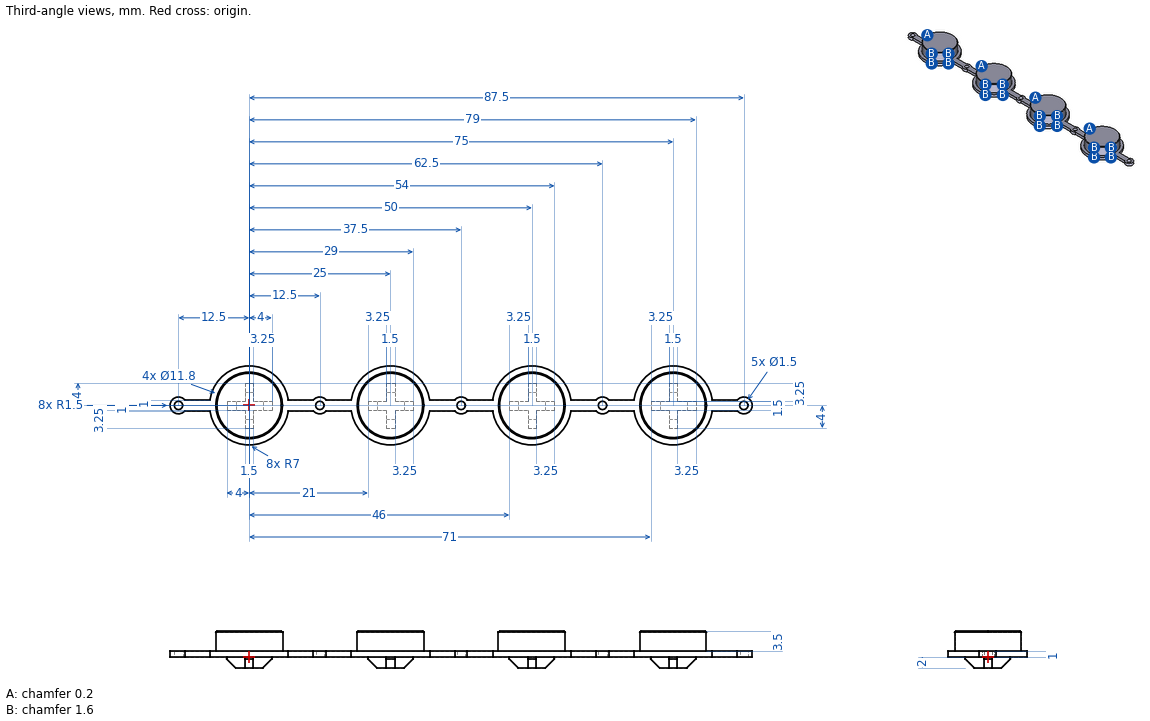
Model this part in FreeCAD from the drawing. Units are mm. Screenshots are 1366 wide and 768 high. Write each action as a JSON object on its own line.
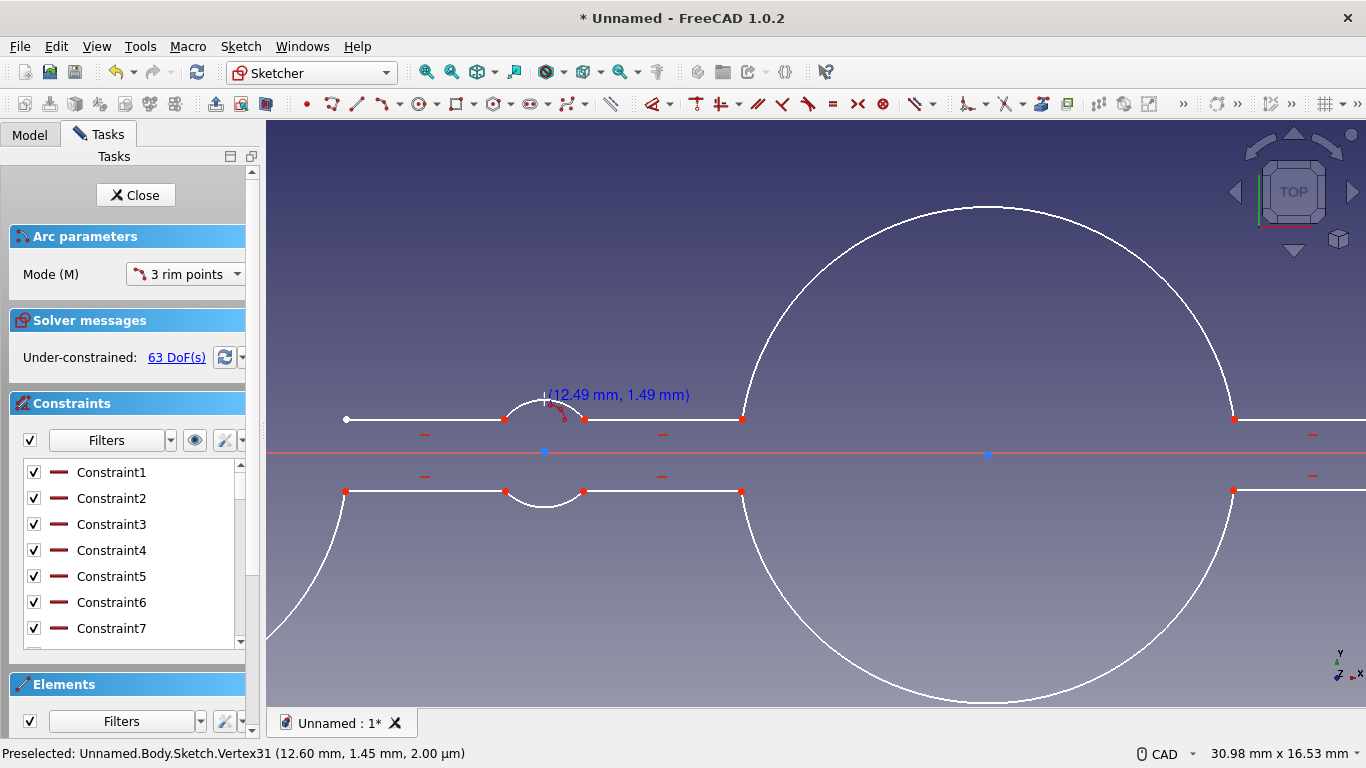
{"action": "left_click", "coordinate": [346, 420]}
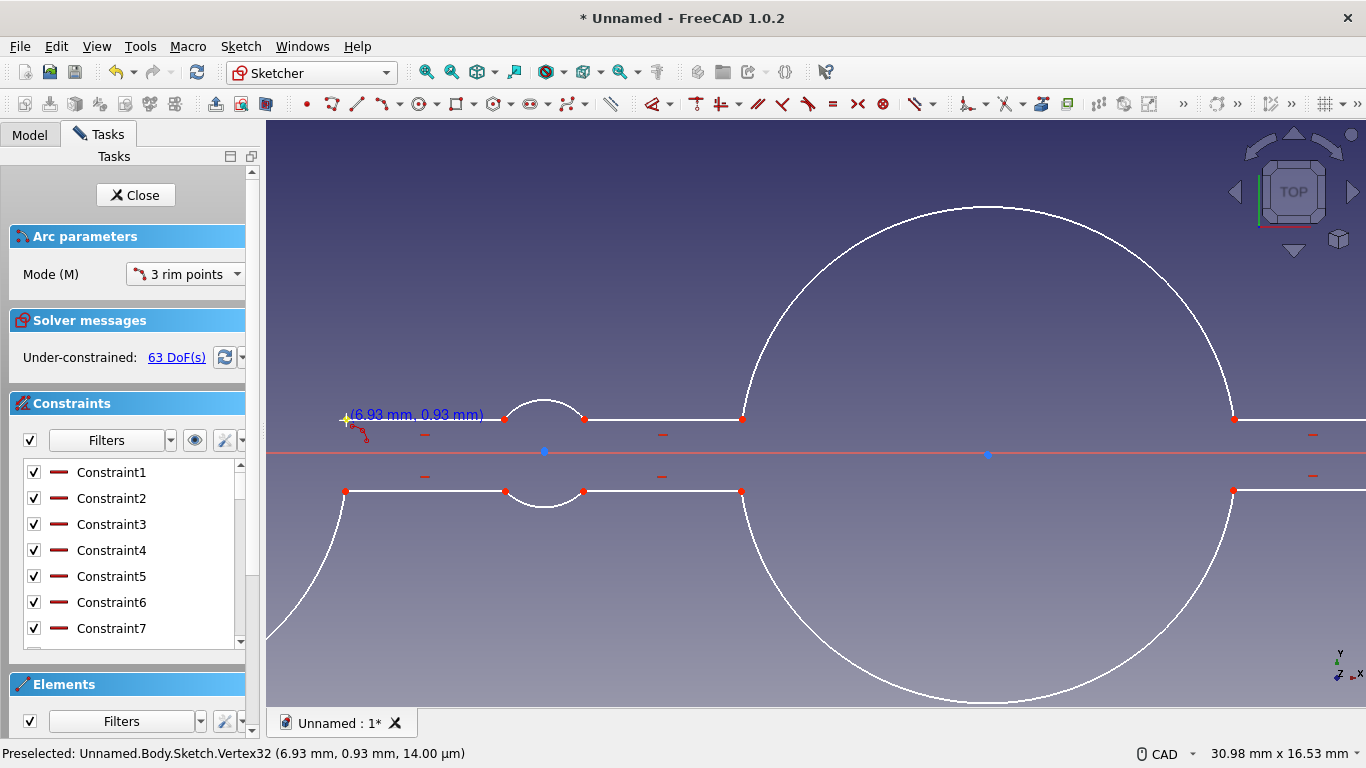
{"action": "scroll", "coordinate": [612, 406], "scroll_direction": "down", "scroll_amount": 9}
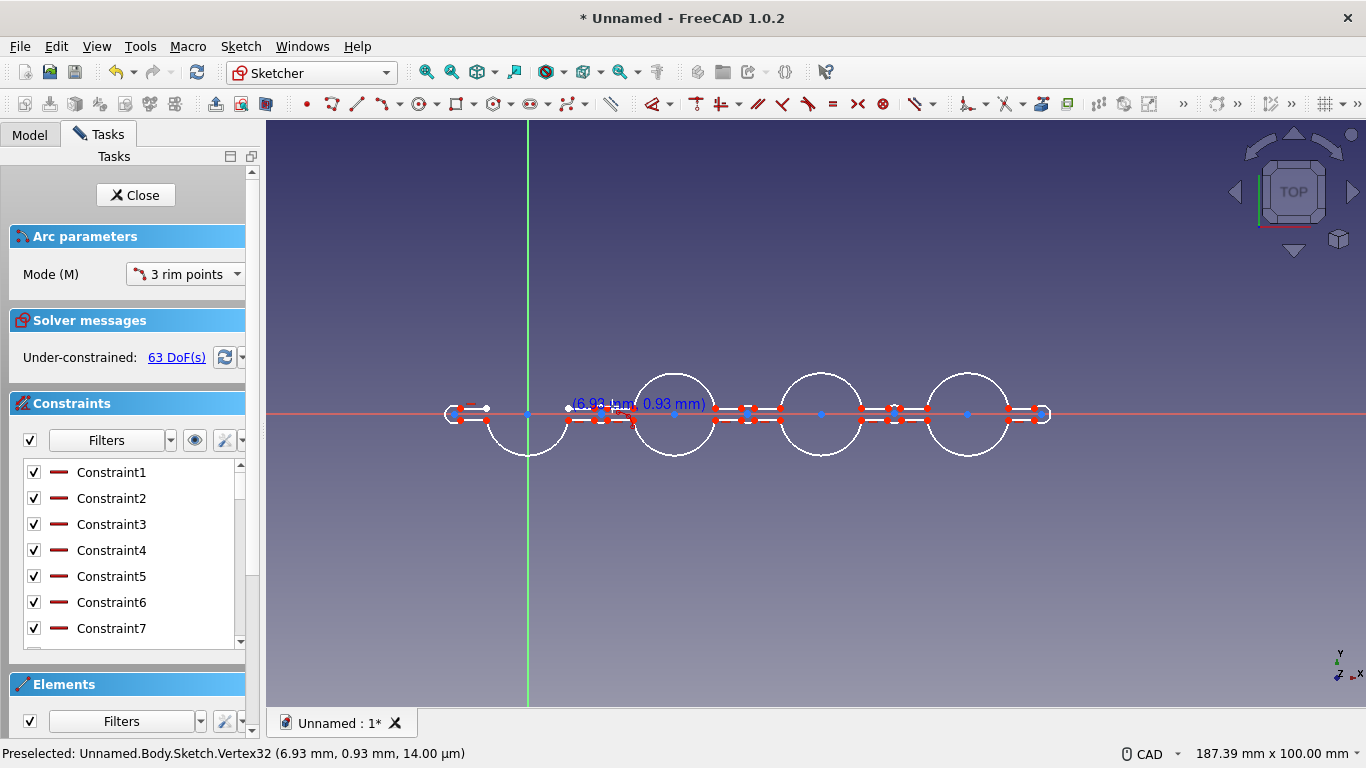
{"action": "scroll", "coordinate": [487, 408], "scroll_direction": "up", "scroll_amount": 5}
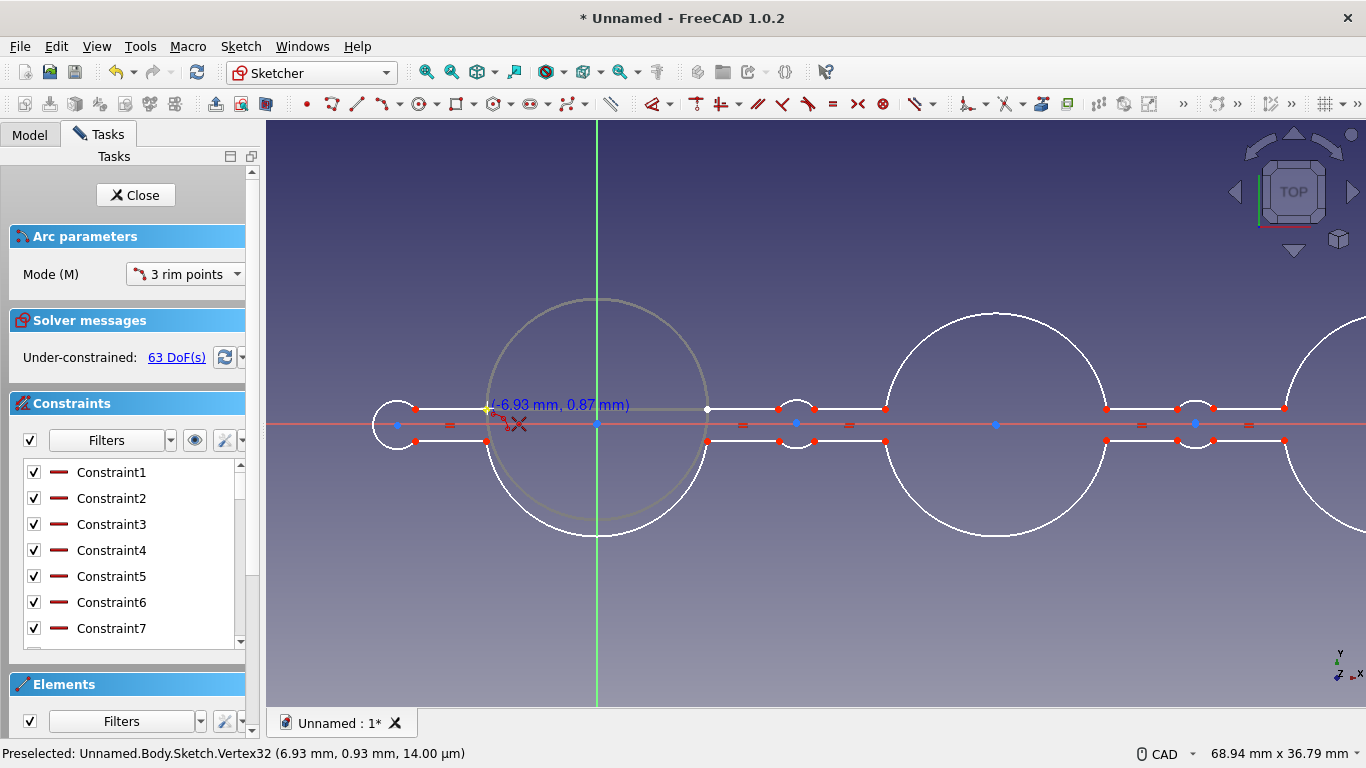
{"action": "left_click", "coordinate": [486, 409]}
{"action": "left_click", "coordinate": [658, 330]}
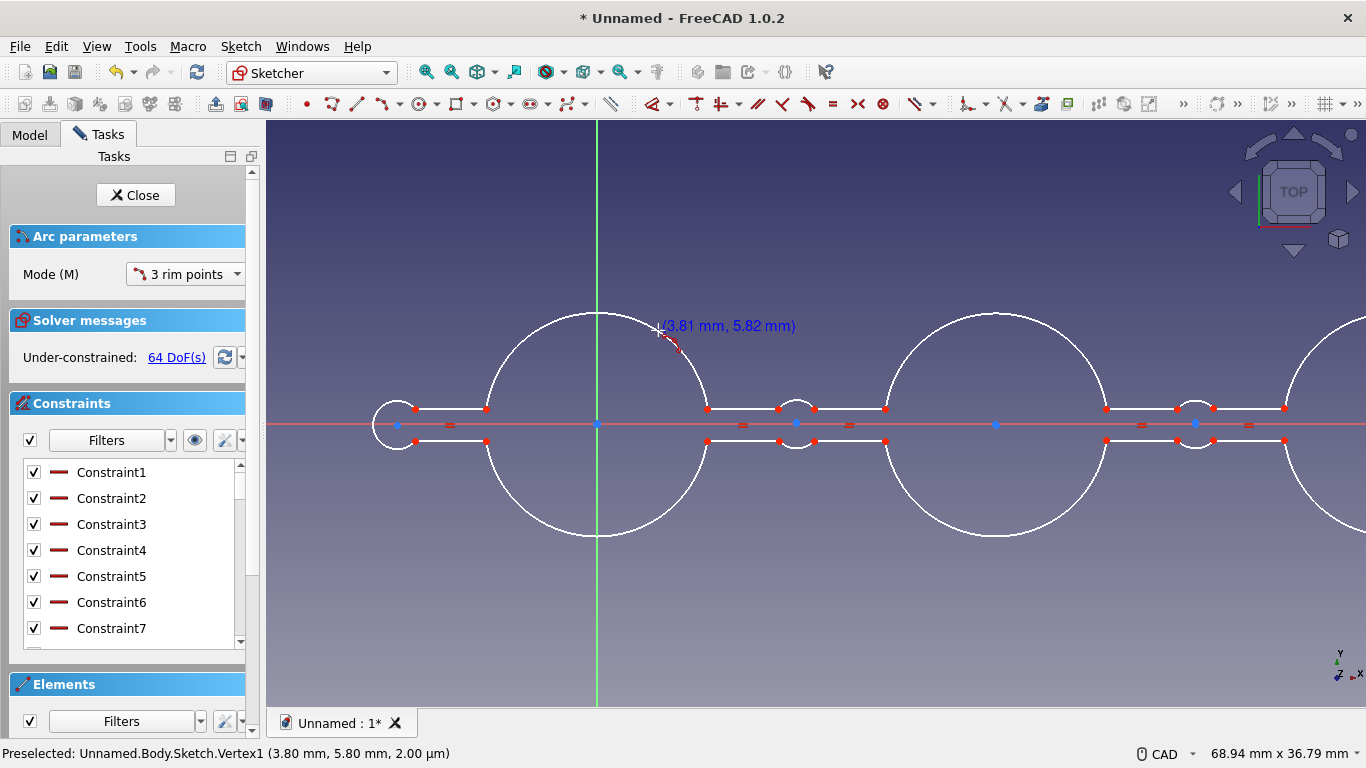
{"action": "key", "text": "g c"}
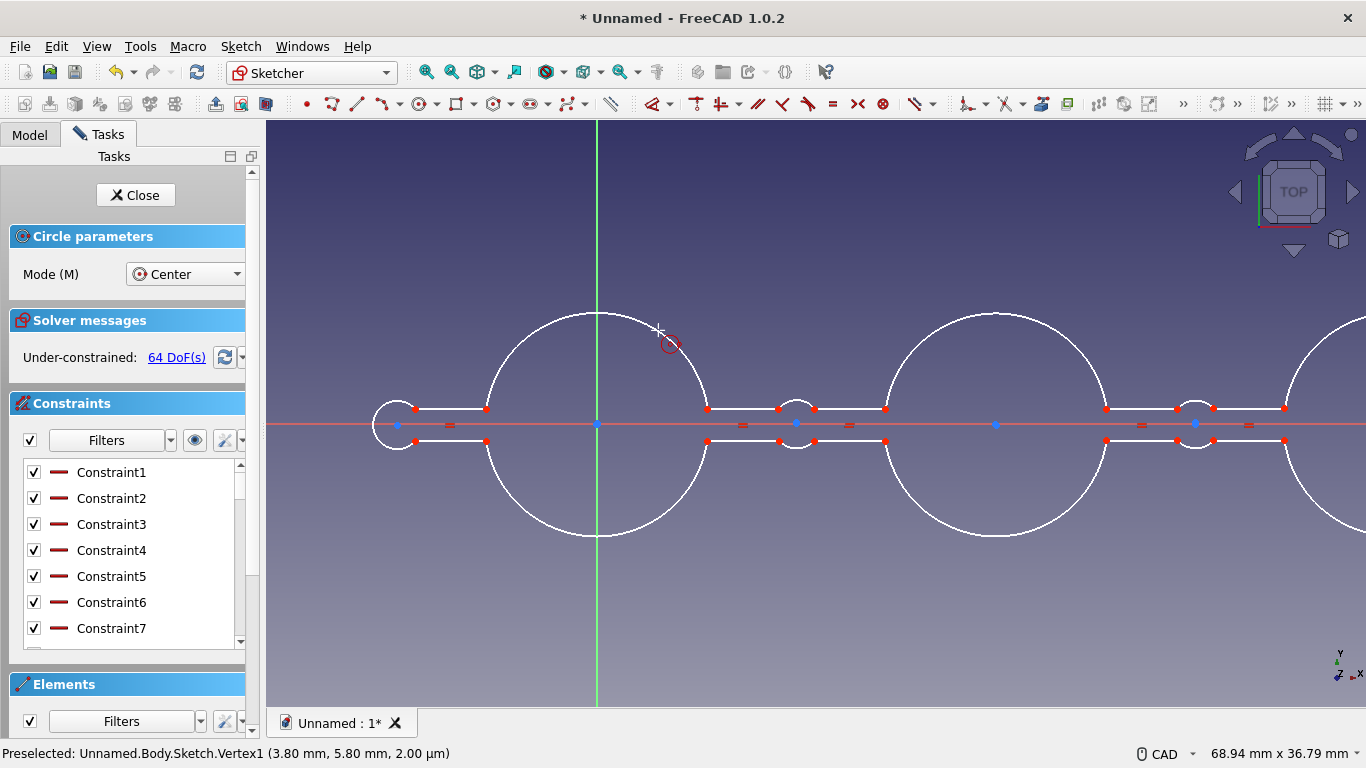
{"action": "scroll", "coordinate": [487, 407], "scroll_direction": "down", "scroll_amount": 5}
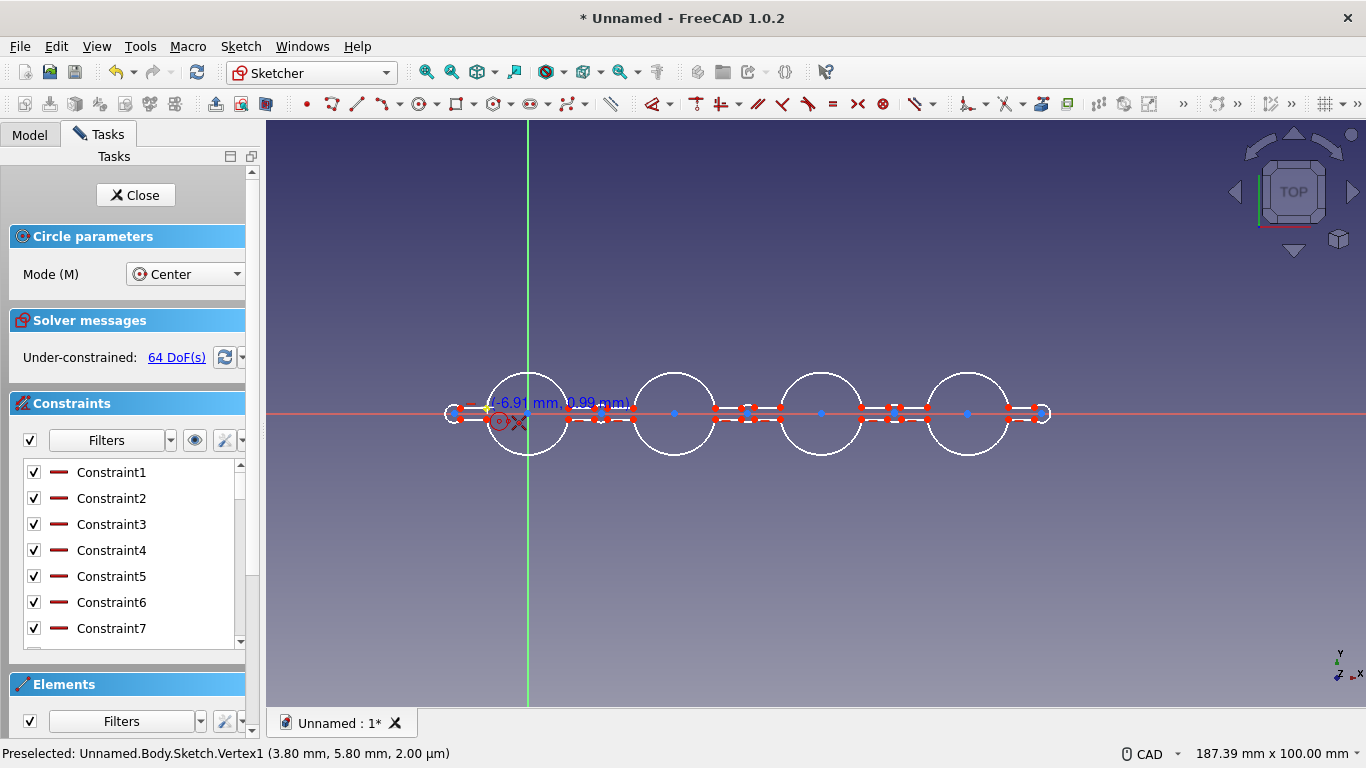
{"action": "scroll", "coordinate": [1041, 414], "scroll_direction": "up", "scroll_amount": 9}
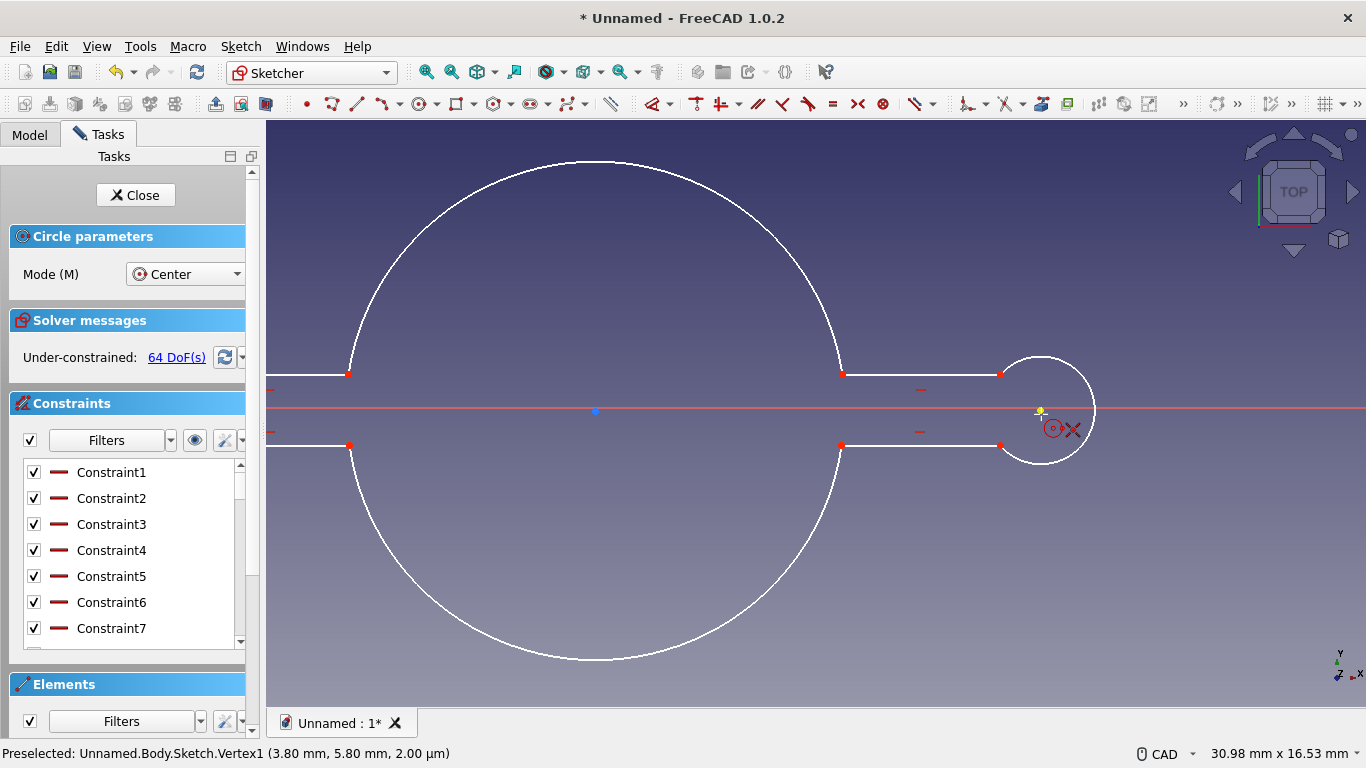
{"action": "scroll", "coordinate": [1041, 414], "scroll_direction": "down", "scroll_amount": 9}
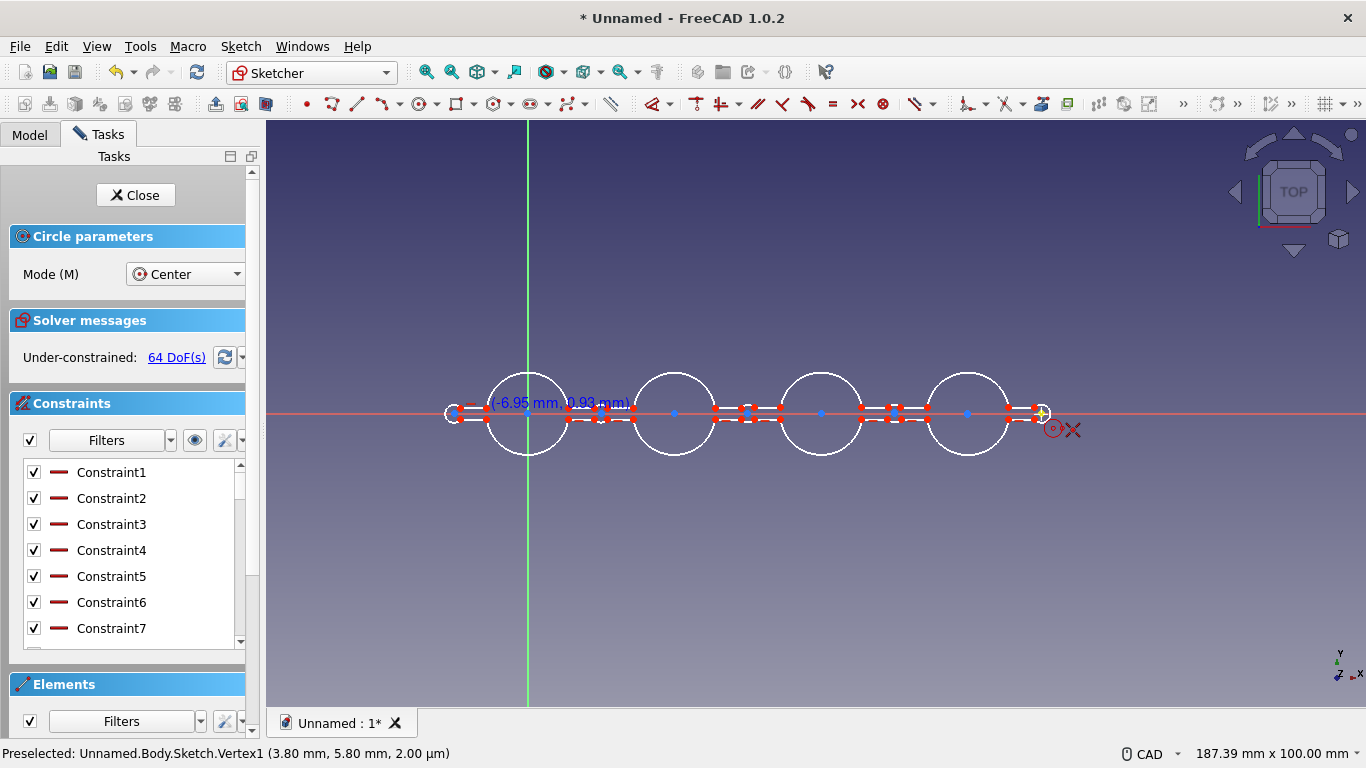
{"action": "scroll", "coordinate": [1041, 414], "scroll_direction": "up", "scroll_amount": 3}